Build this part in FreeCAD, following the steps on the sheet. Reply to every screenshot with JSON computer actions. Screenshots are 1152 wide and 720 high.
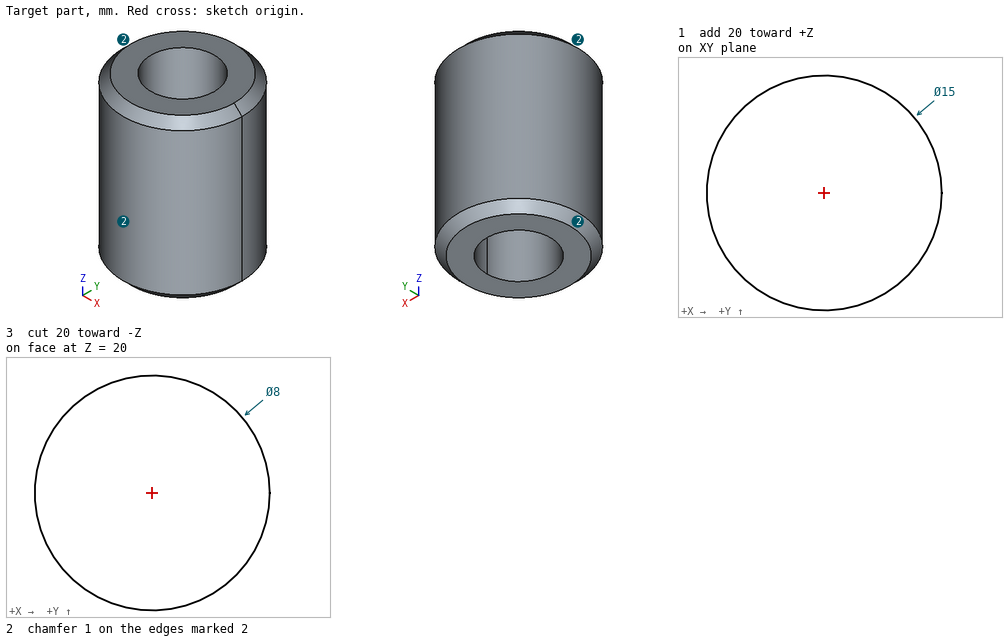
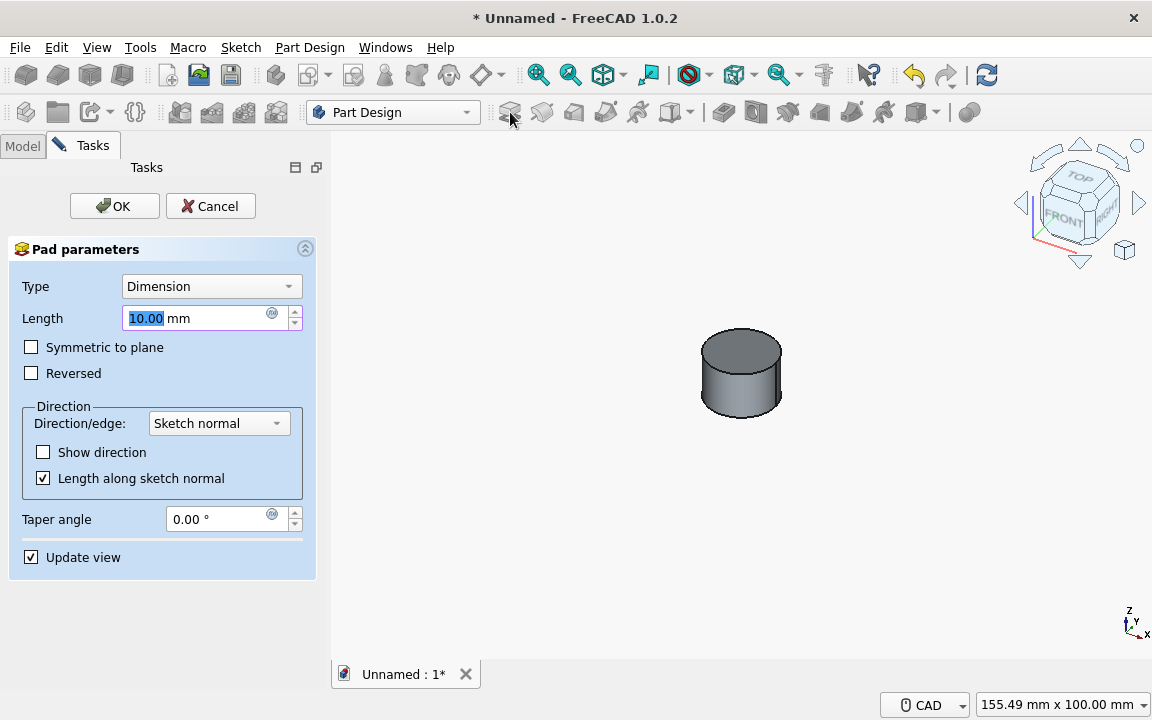
{"action": "type", "text": "20"}
{"action": "key", "text": "Tab"}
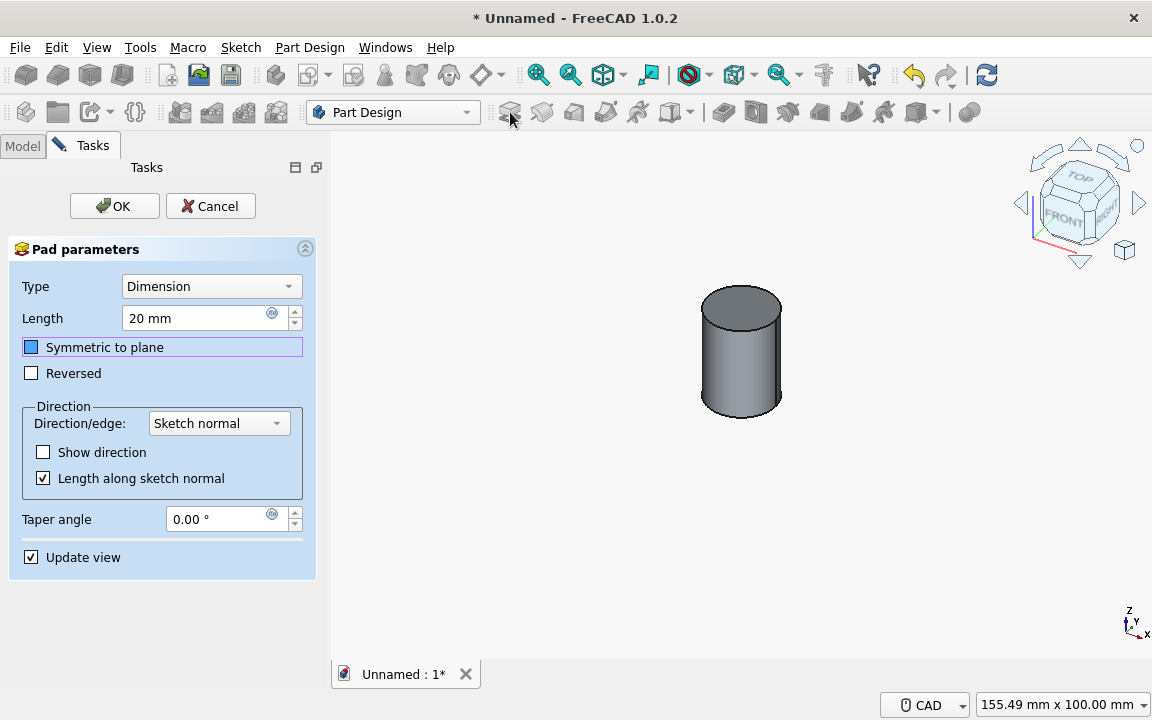
{"action": "left_click", "coordinate": [115, 206]}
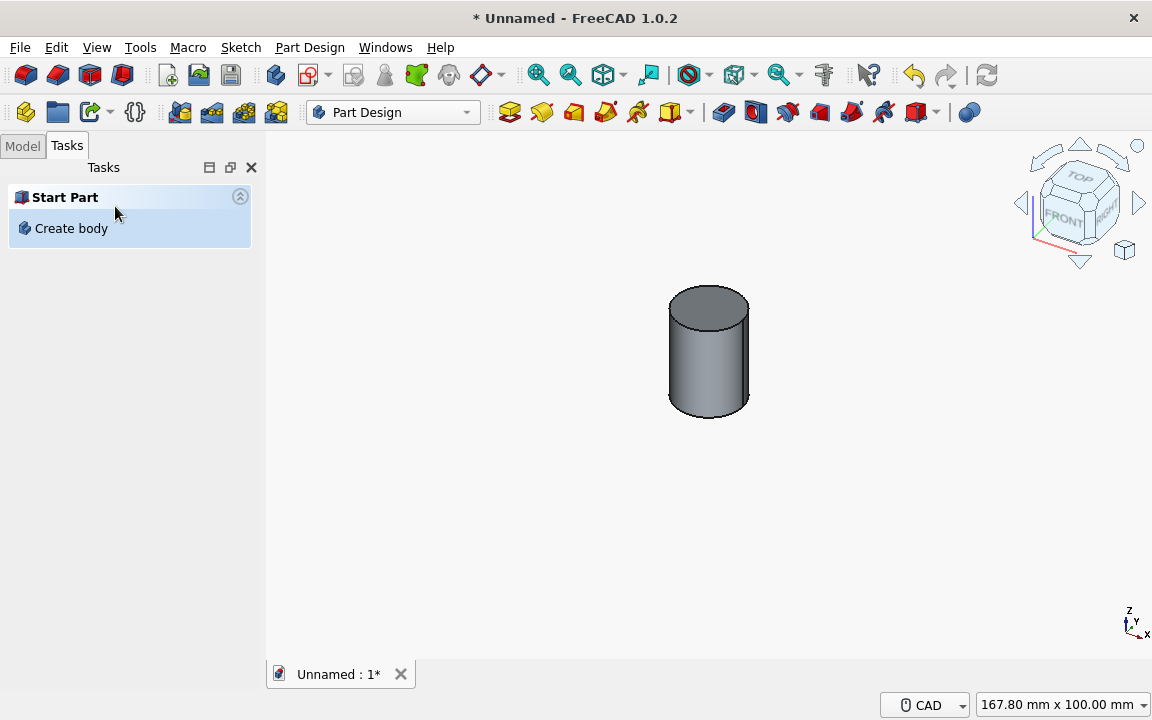
{"action": "left_click", "coordinate": [540, 76]}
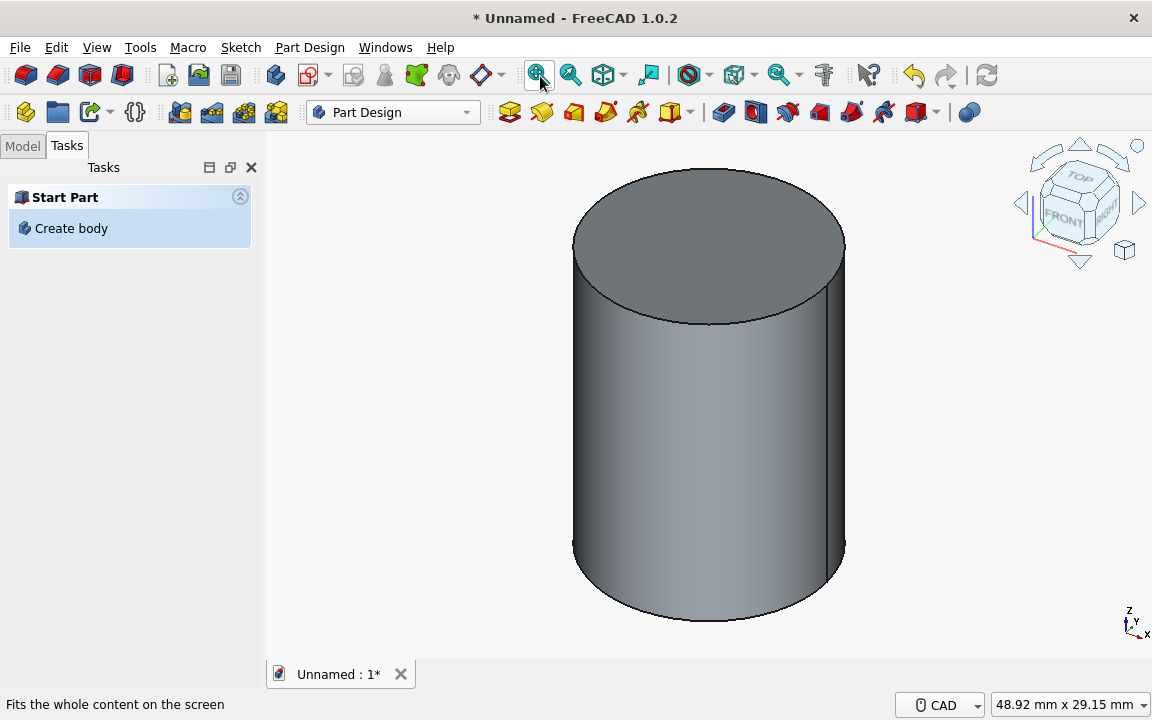
{"action": "left_click", "coordinate": [574, 254]}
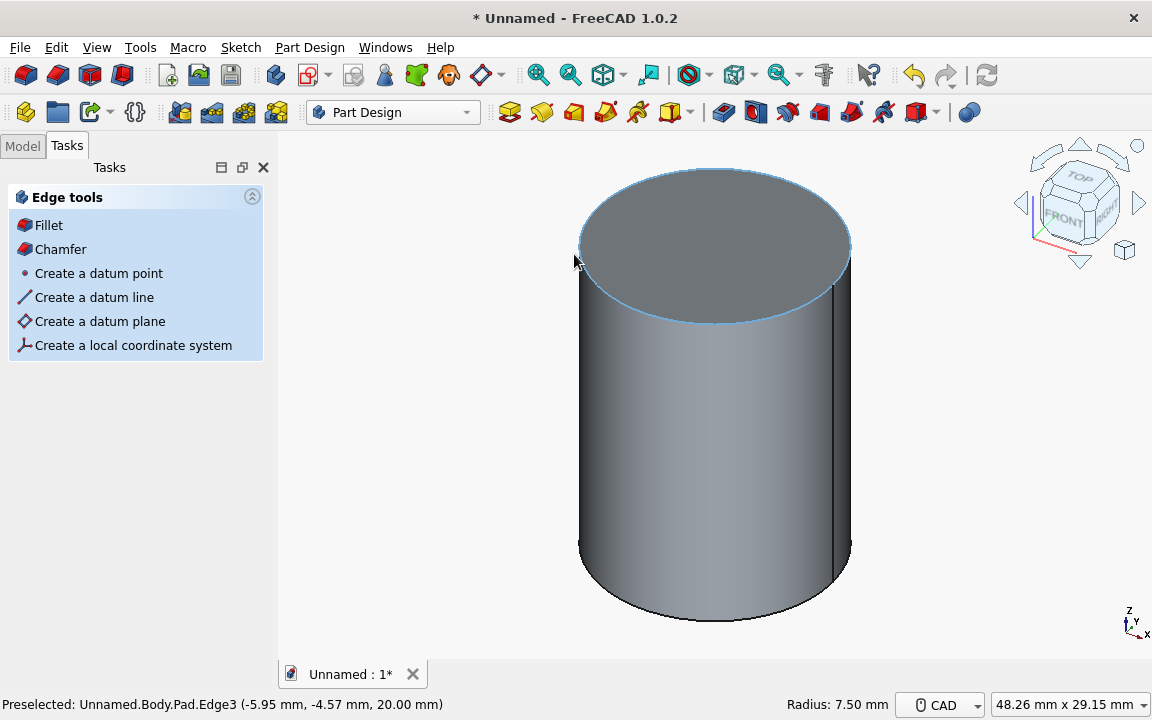
{"action": "key", "text": "0"}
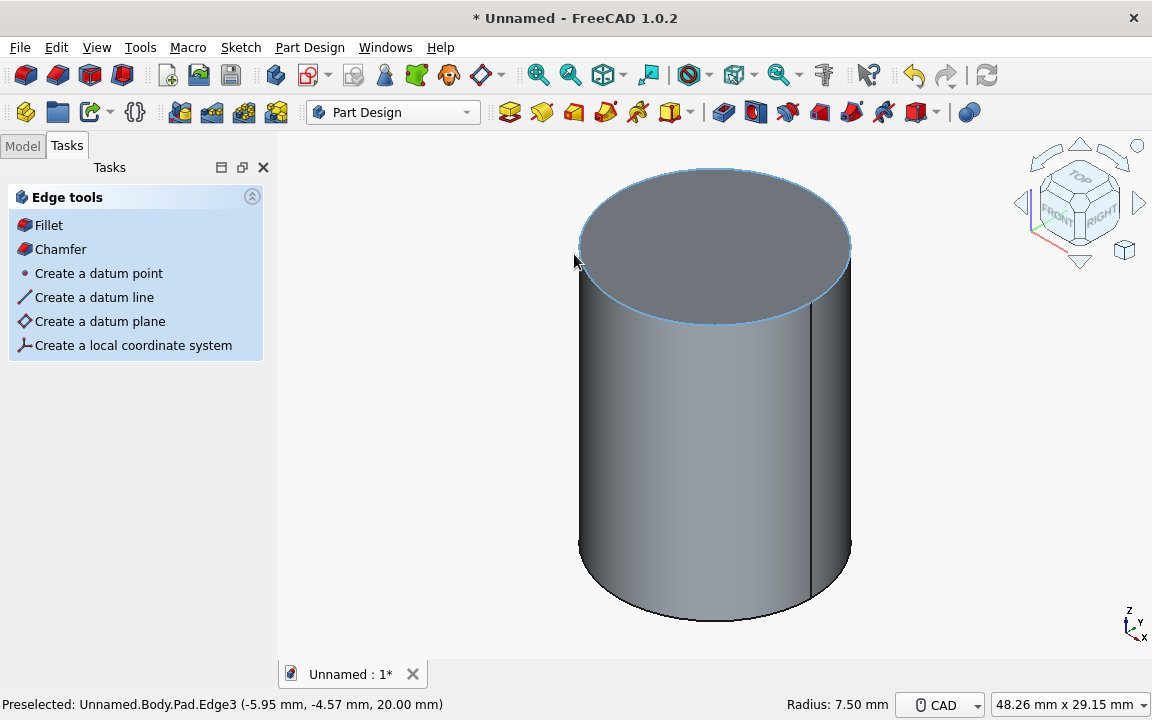
{"action": "key", "text": "2"}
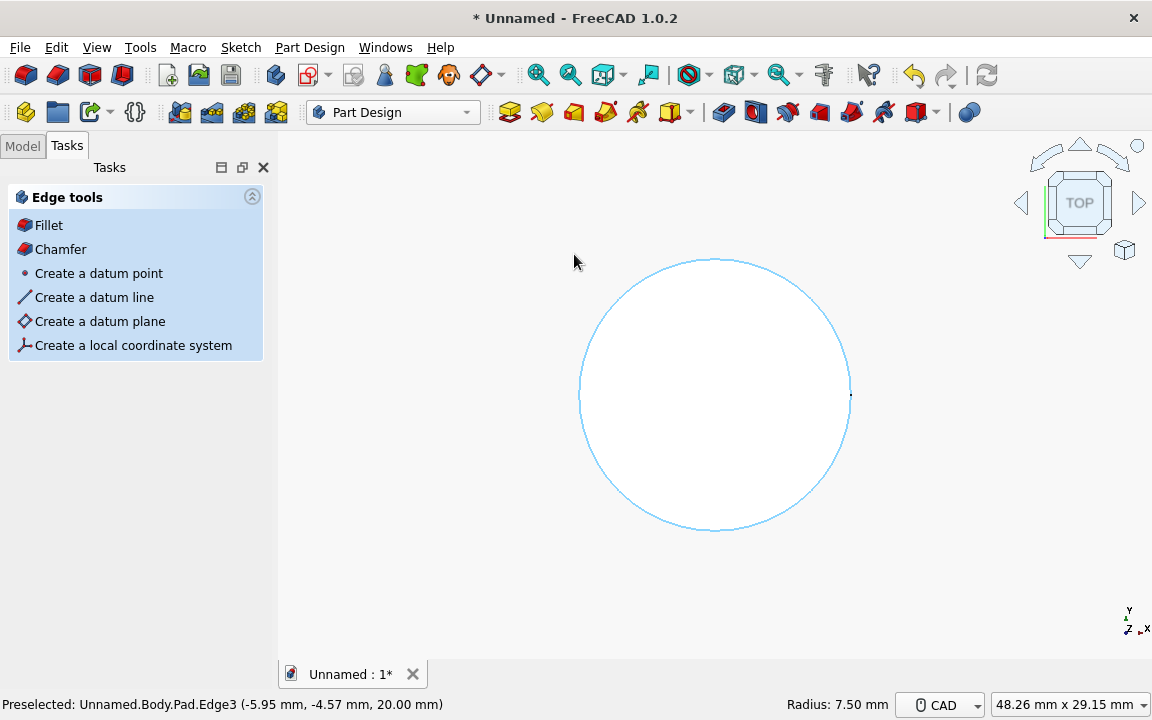
{"action": "key", "text": "1"}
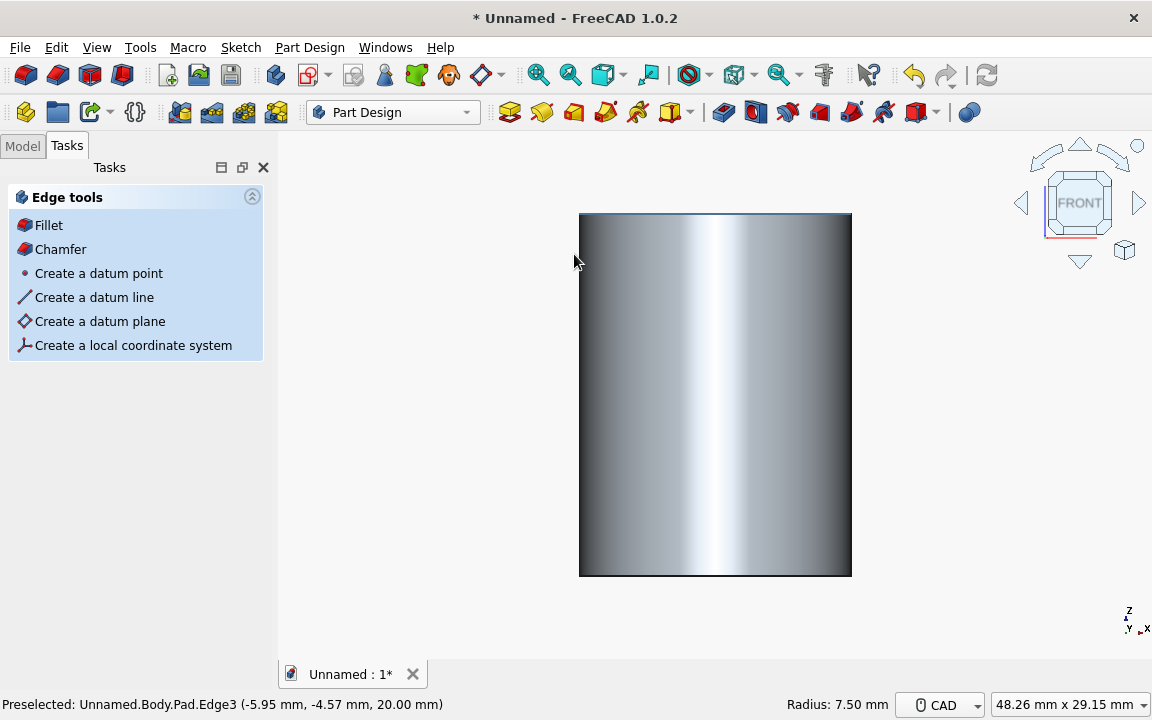
{"action": "left_click", "coordinate": [605, 575], "text": "ctrl"}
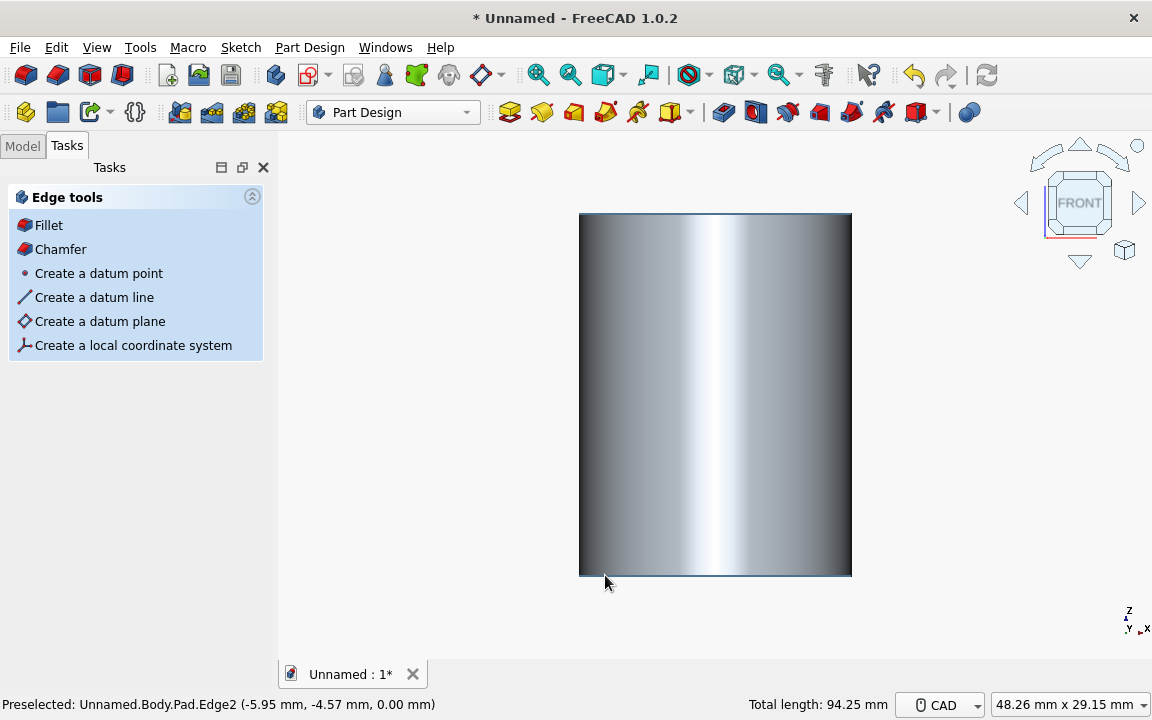
{"action": "left_click", "coordinate": [58, 76]}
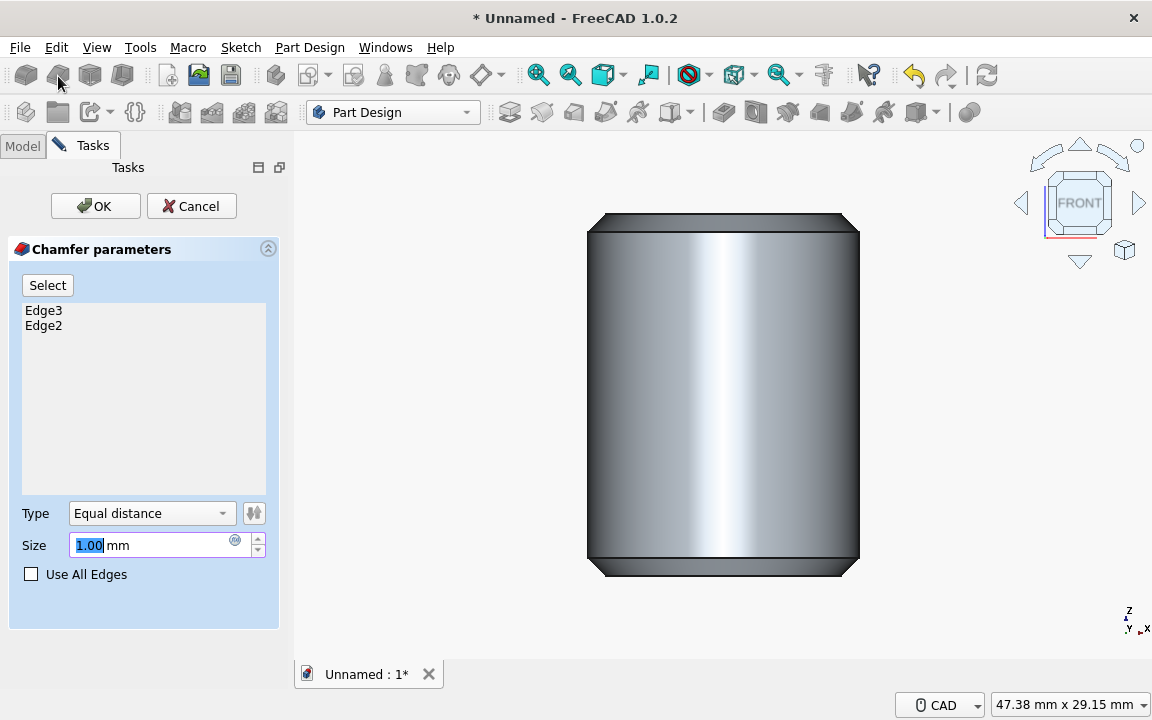
{"action": "type", "text": "1"}
{"action": "key", "text": "Tab"}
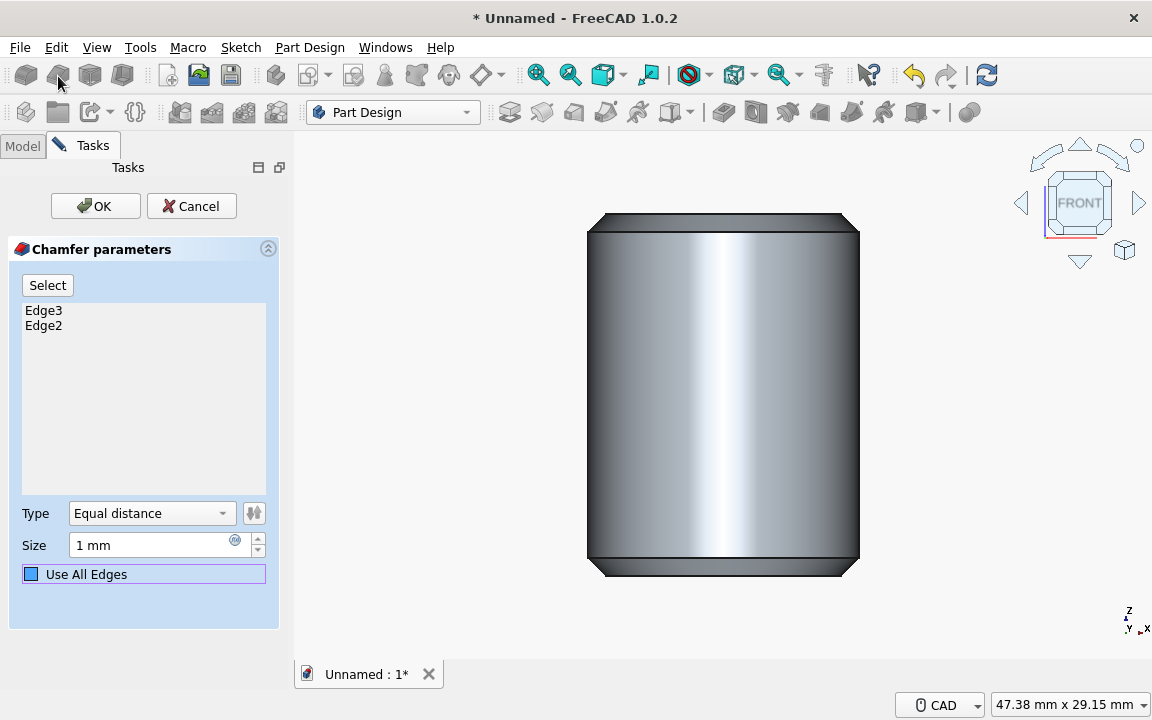
{"action": "left_click", "coordinate": [96, 206]}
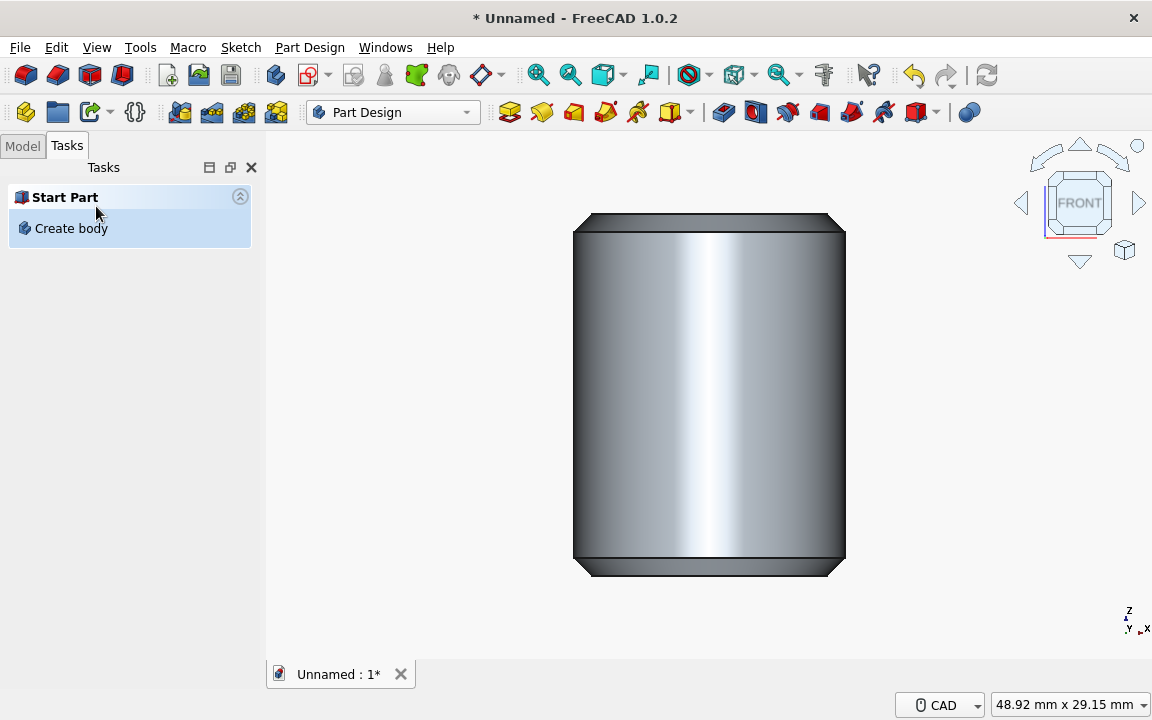
{"action": "key", "text": "0"}